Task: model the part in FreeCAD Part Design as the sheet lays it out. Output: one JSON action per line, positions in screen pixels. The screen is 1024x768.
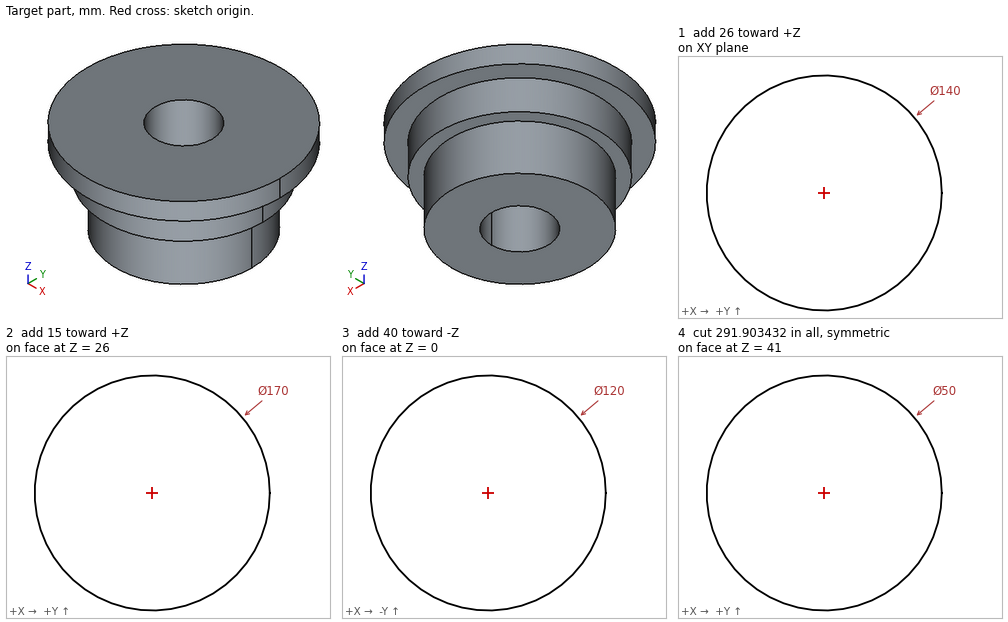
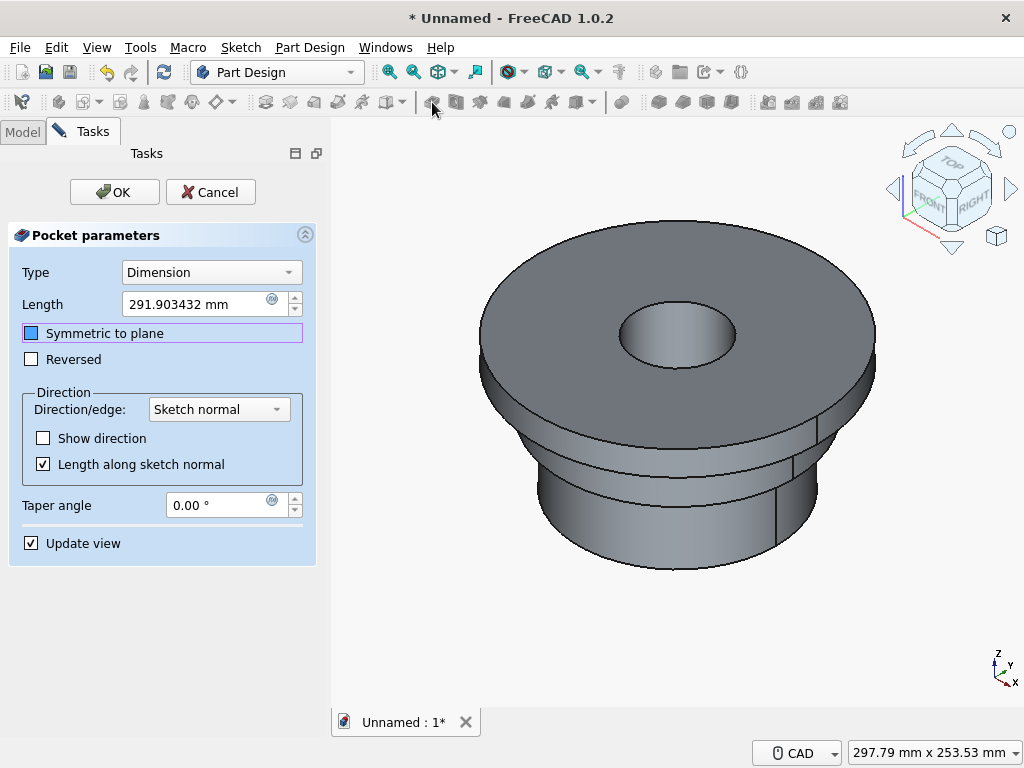
{"action": "left_click", "coordinate": [30, 333]}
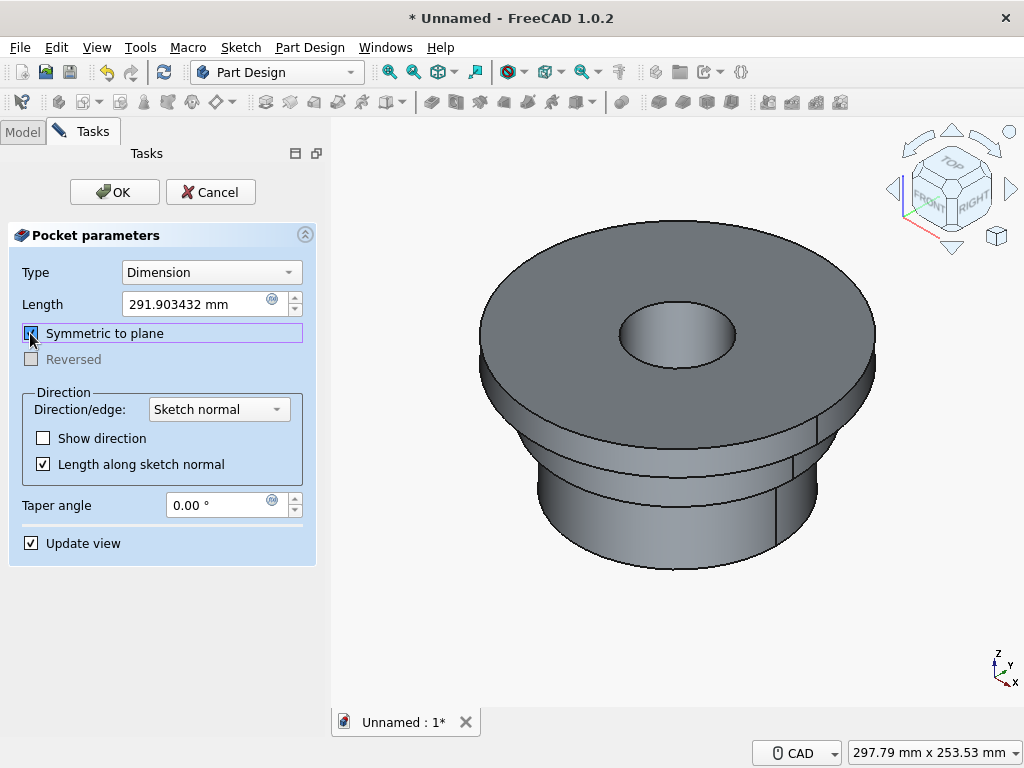
{"action": "left_click", "coordinate": [115, 192]}